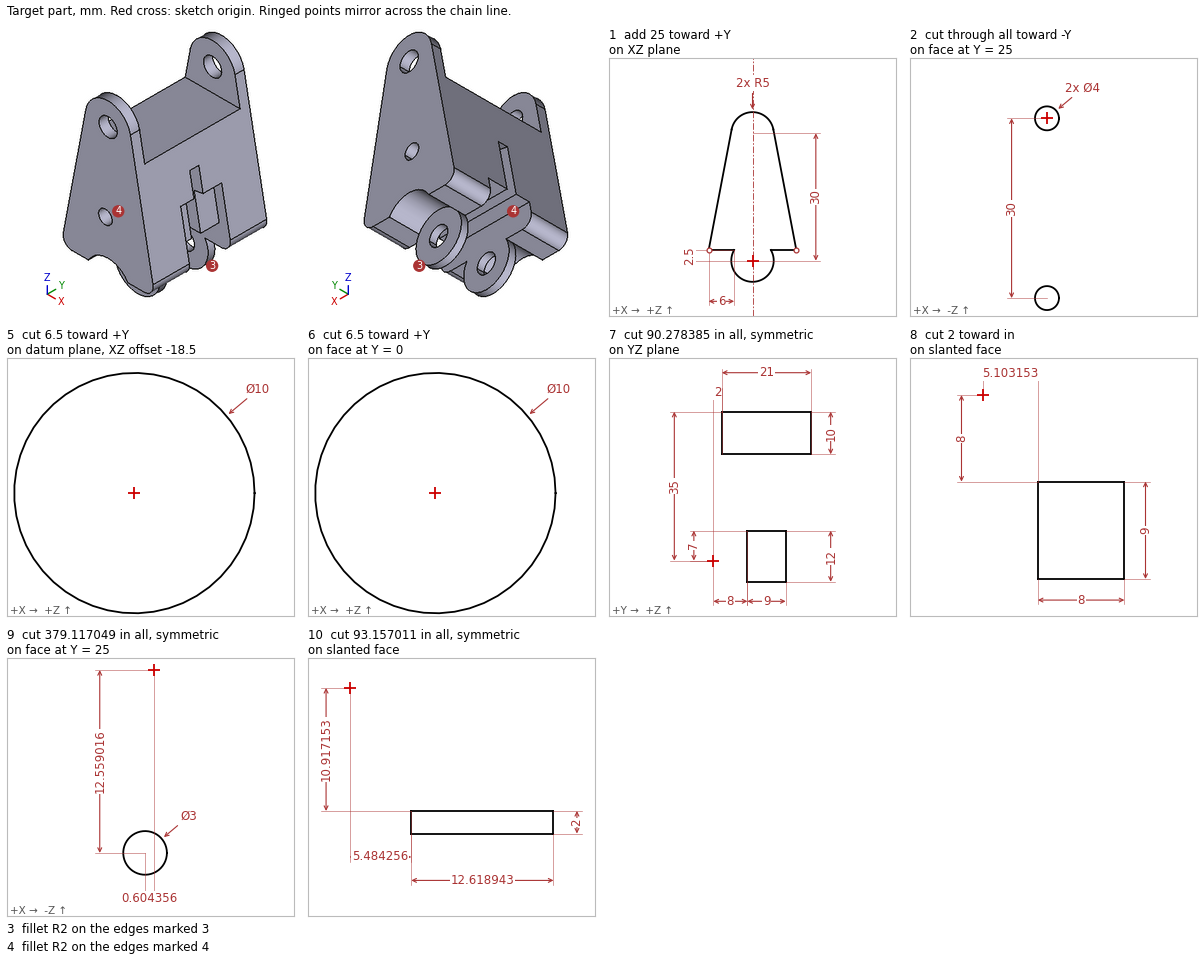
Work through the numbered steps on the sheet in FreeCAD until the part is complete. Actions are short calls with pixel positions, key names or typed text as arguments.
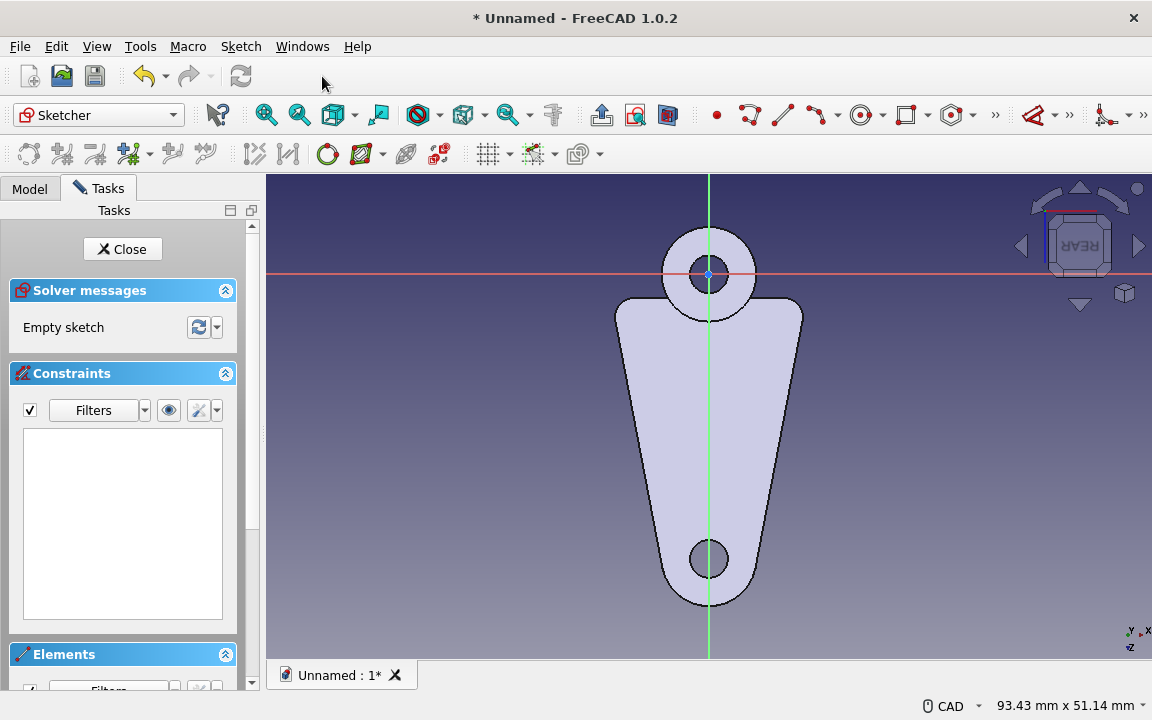
scroll(709, 391, up, 12)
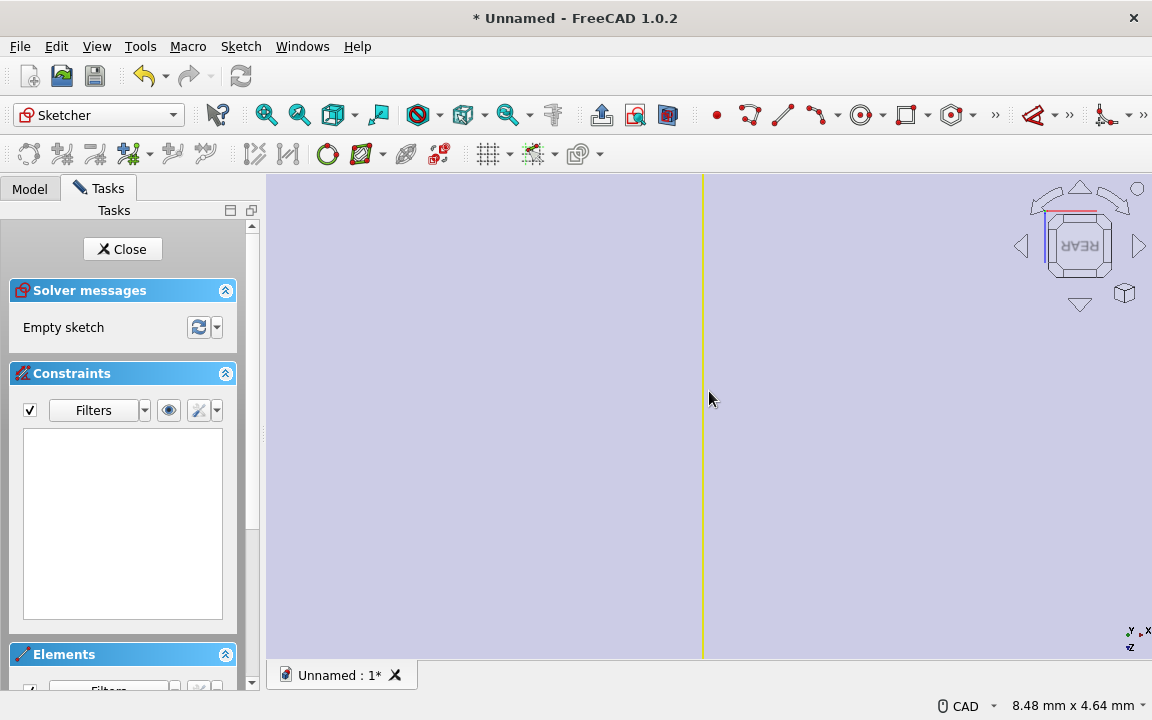
key(g)
key(c)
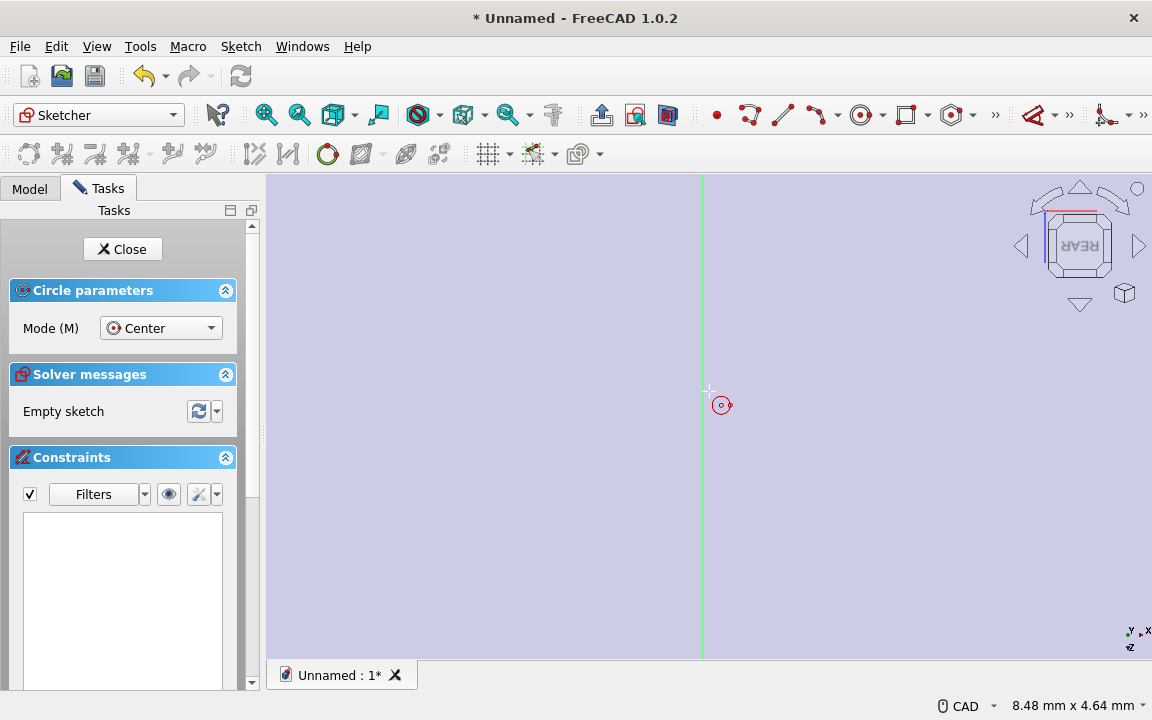
click(640, 413)
move(751, 303)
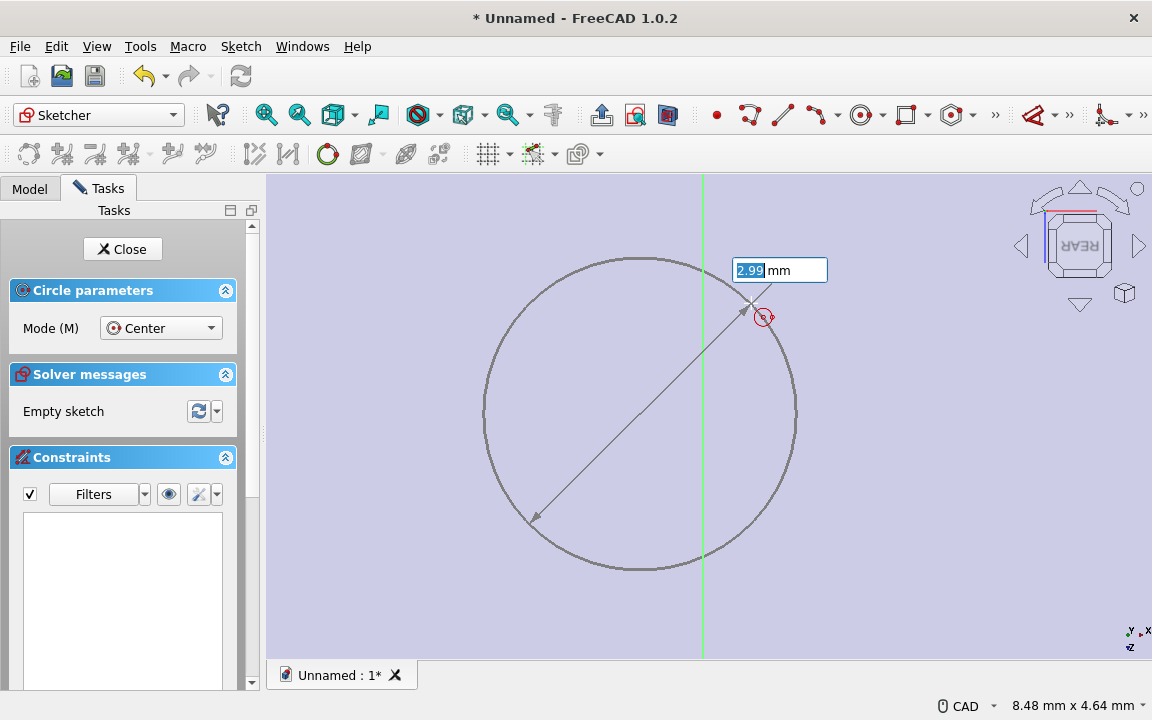
text(3)
key(Return)
key(Escape)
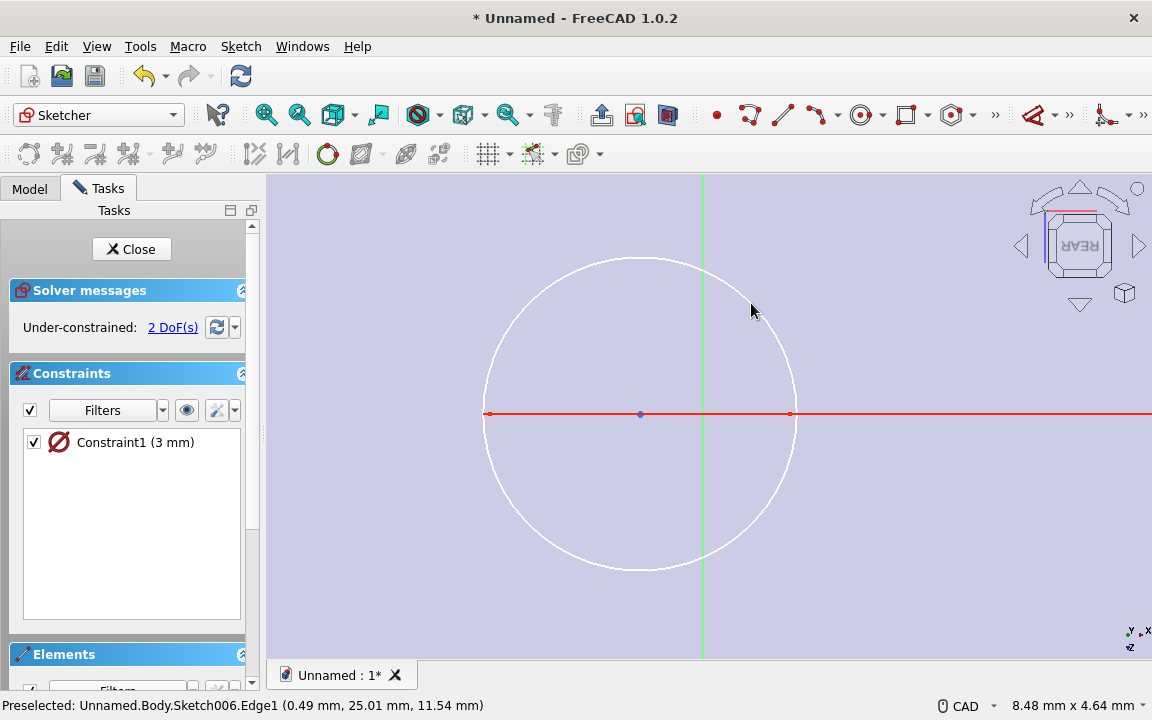
key(d)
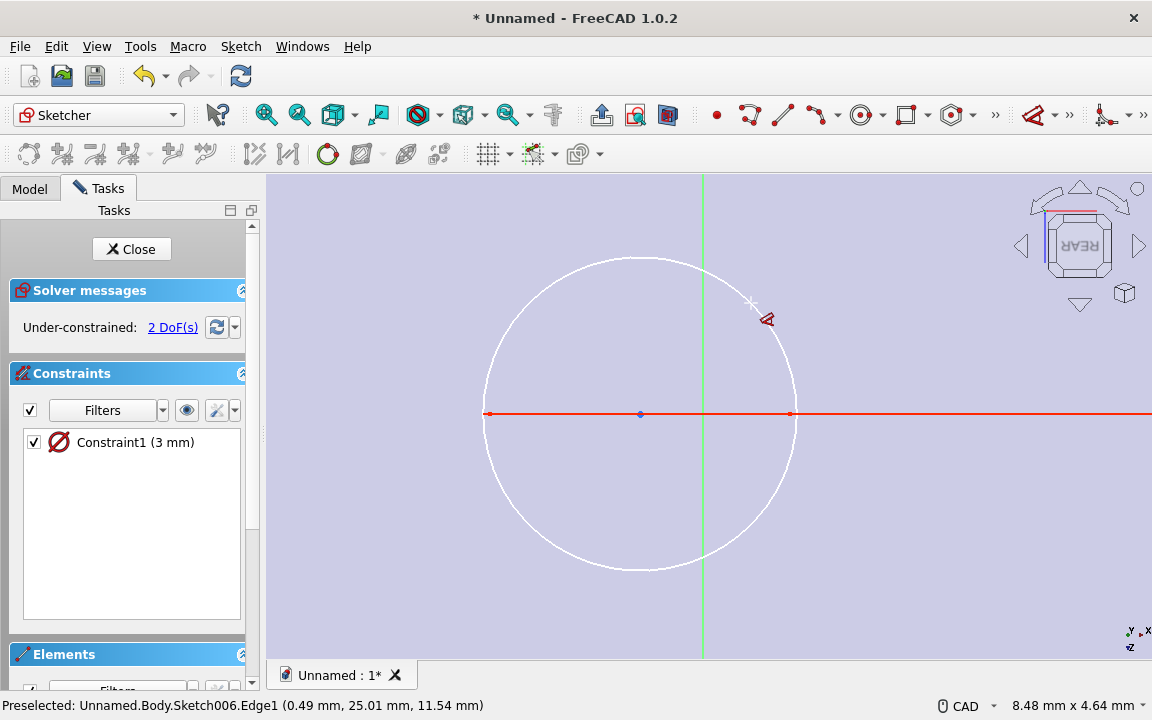
click(640, 414)
click(672, 448)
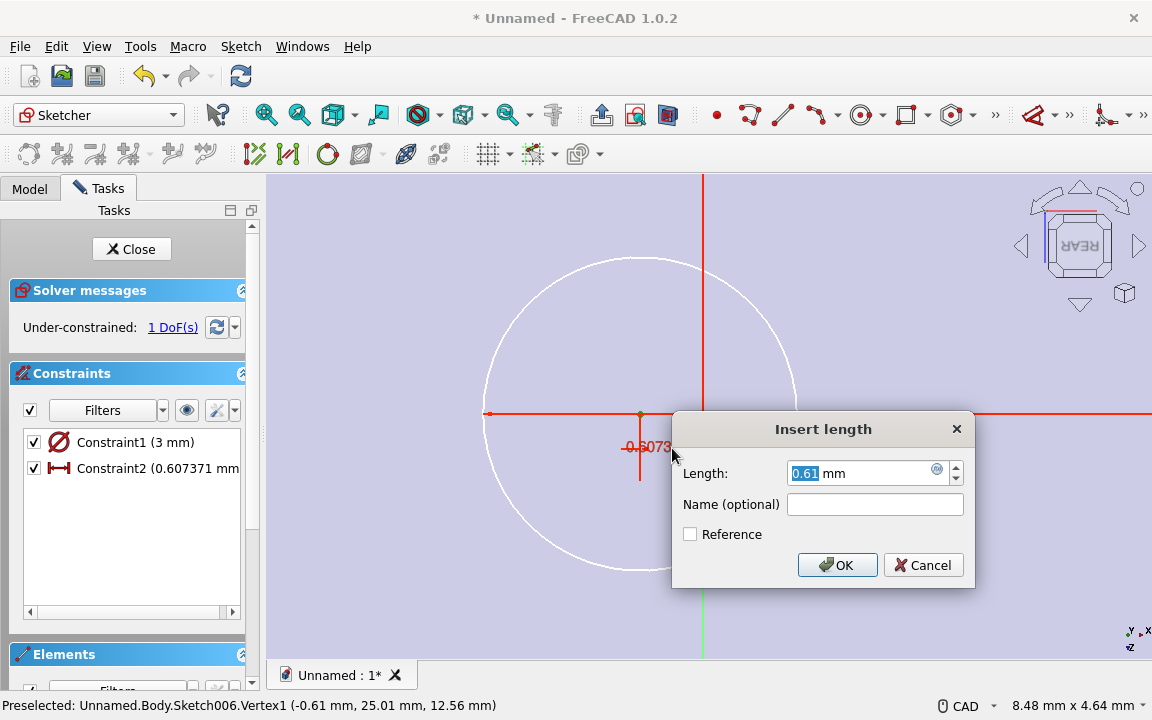
text(0.604356)
key(Return)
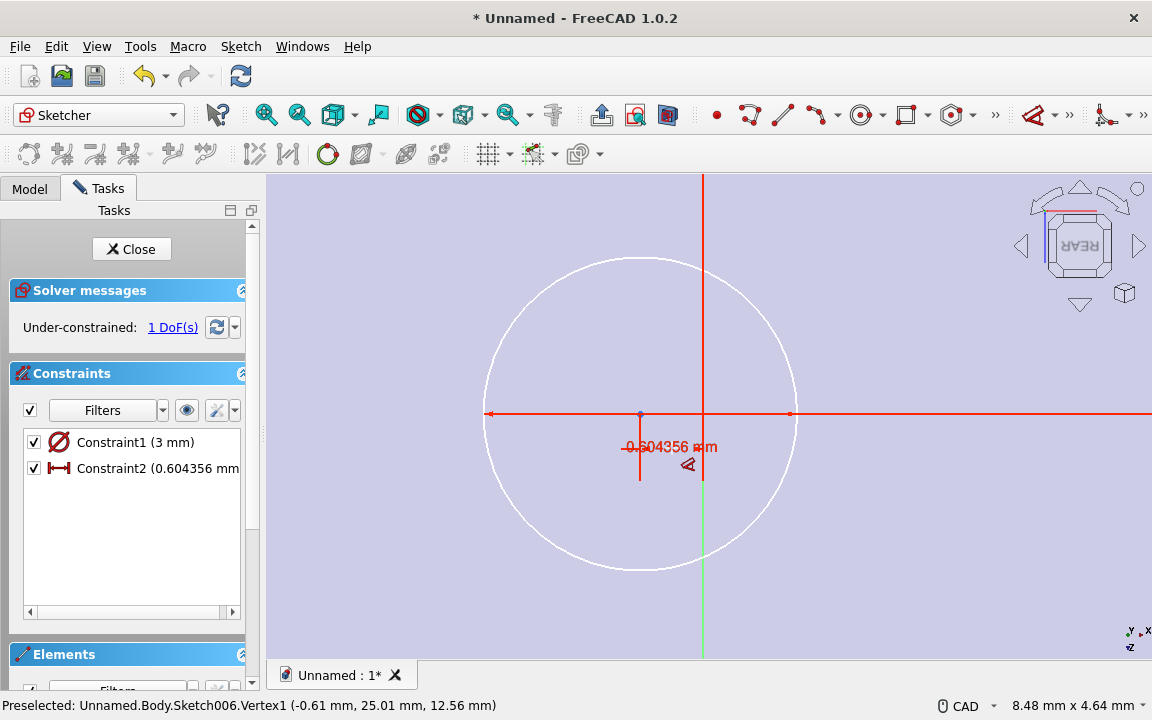
click(640, 414)
click(737, 259)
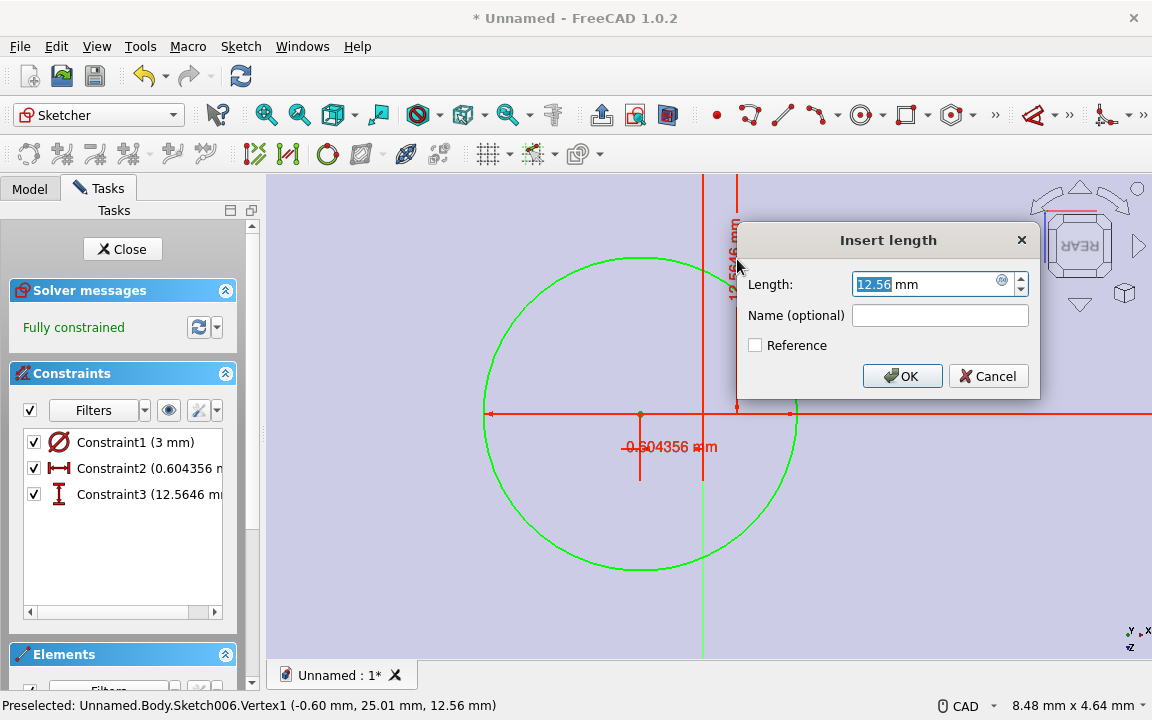
text(12.559016)
key(Return)
key(Escape)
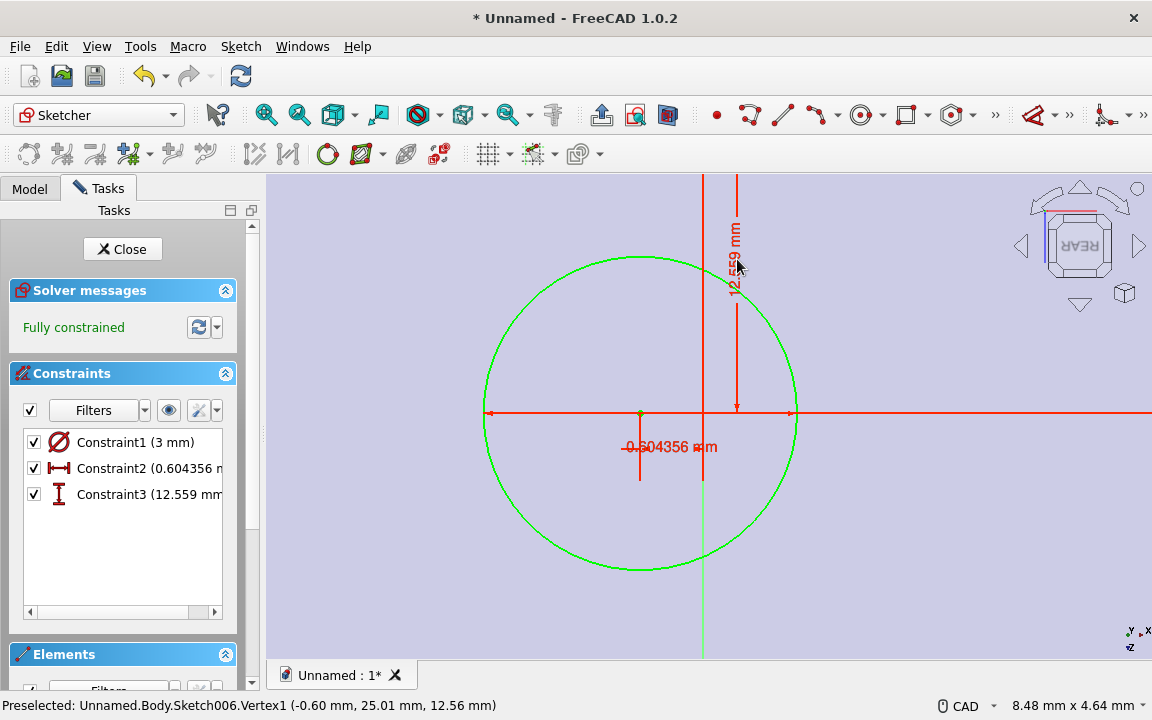
click(123, 249)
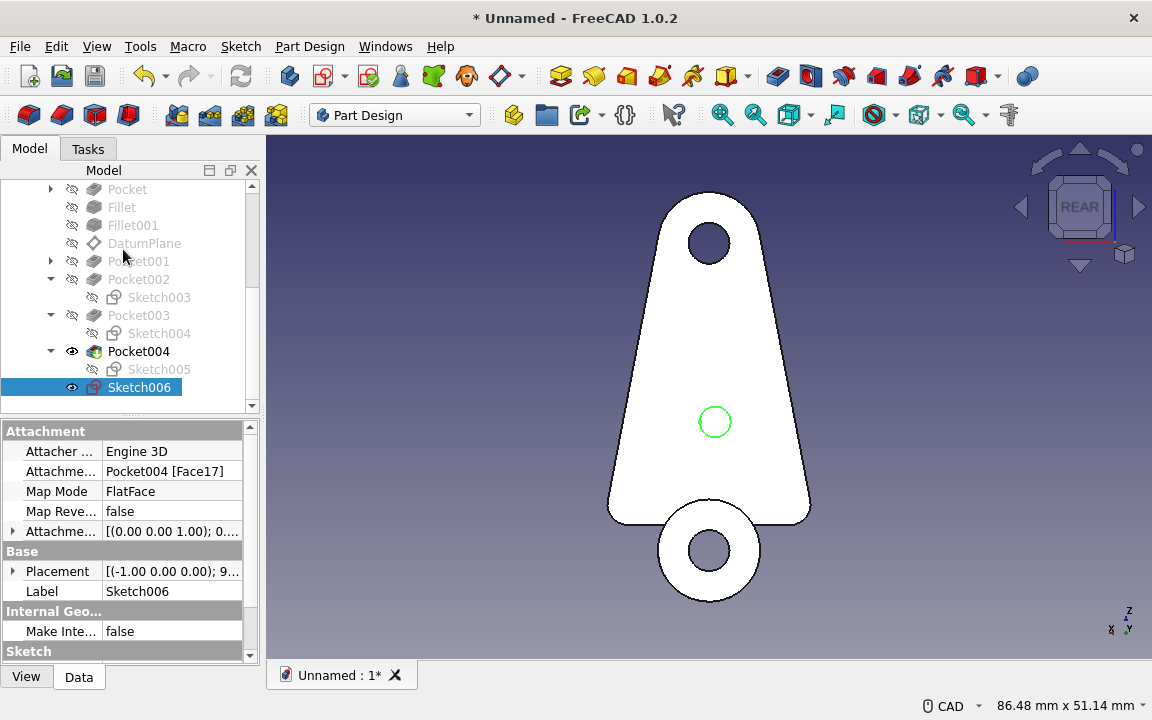
click(778, 76)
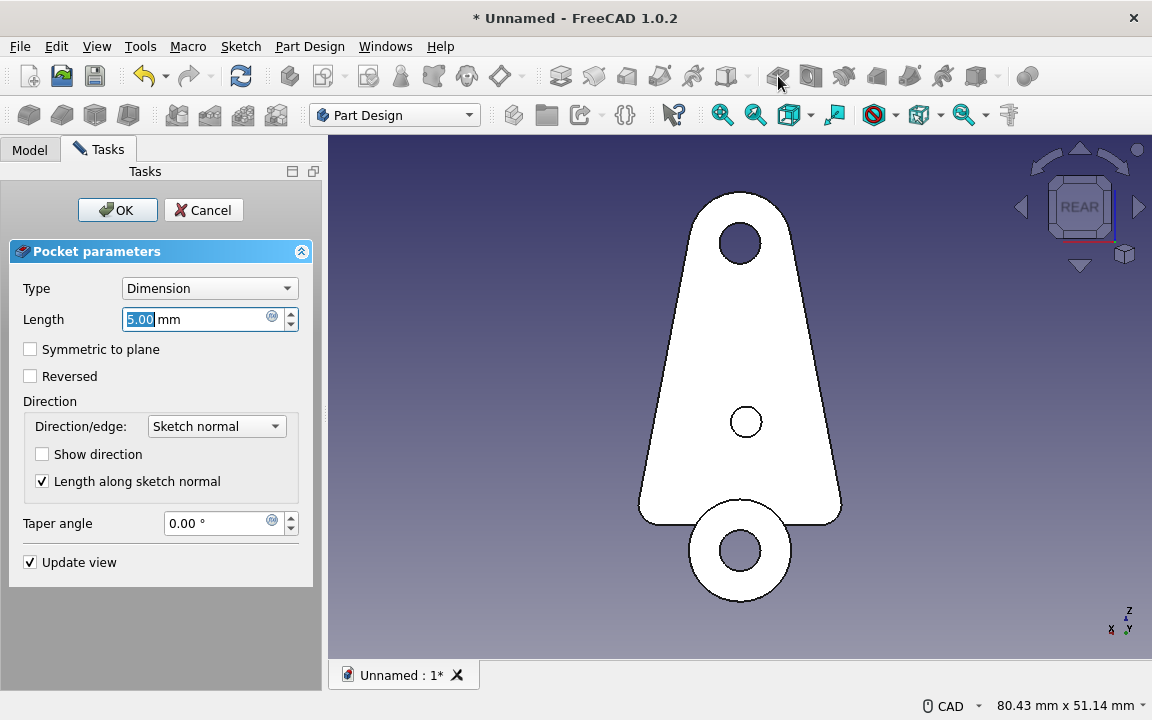
text(379.117049)
key(Tab)